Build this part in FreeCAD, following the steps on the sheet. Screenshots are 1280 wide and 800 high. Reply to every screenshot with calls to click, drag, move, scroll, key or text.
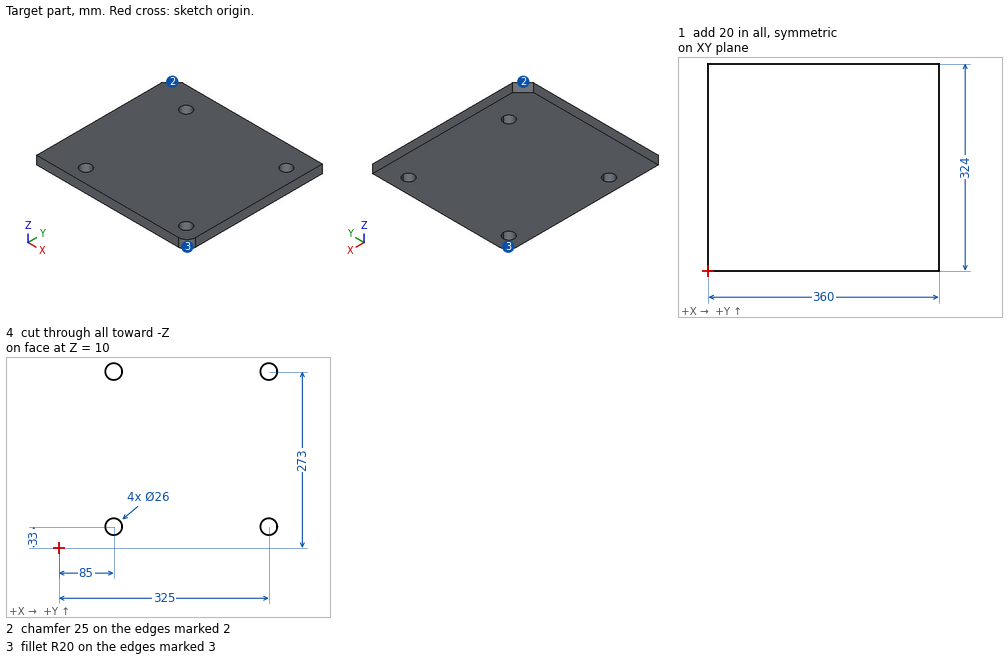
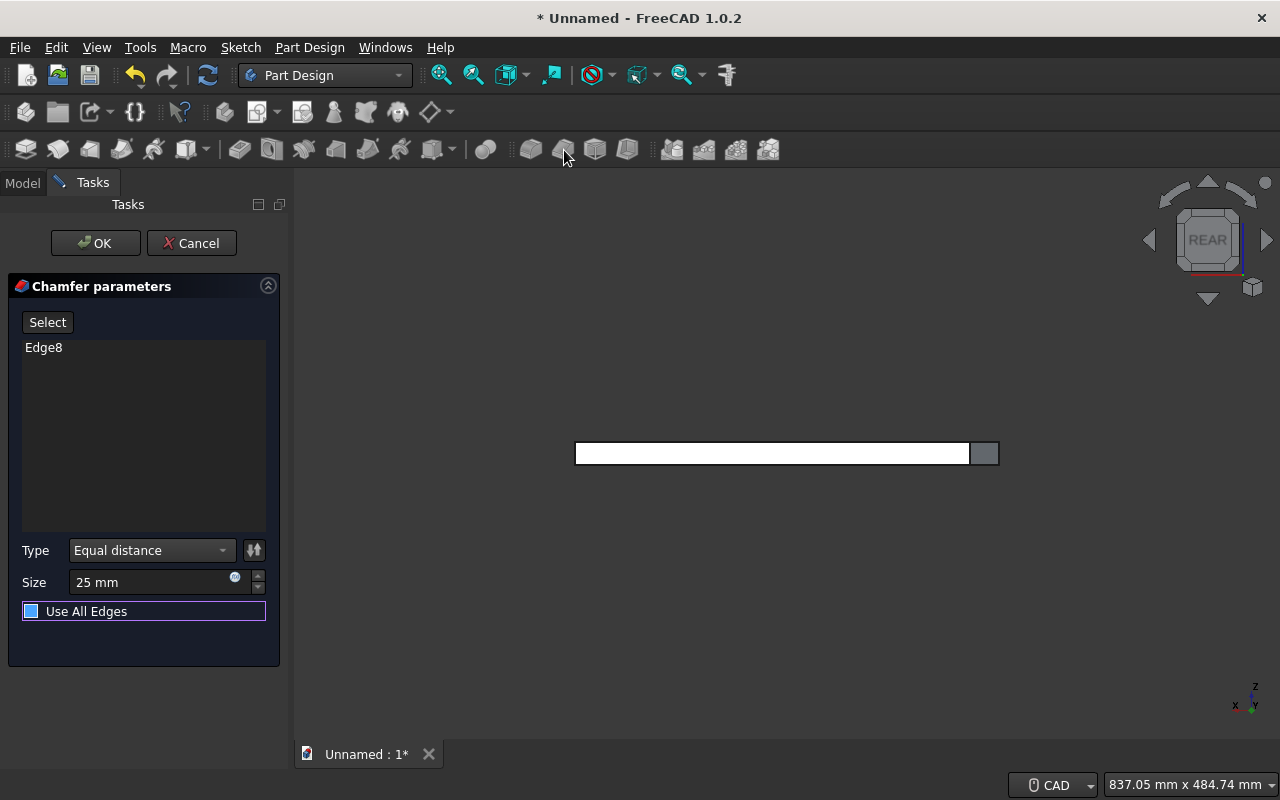
click(96, 243)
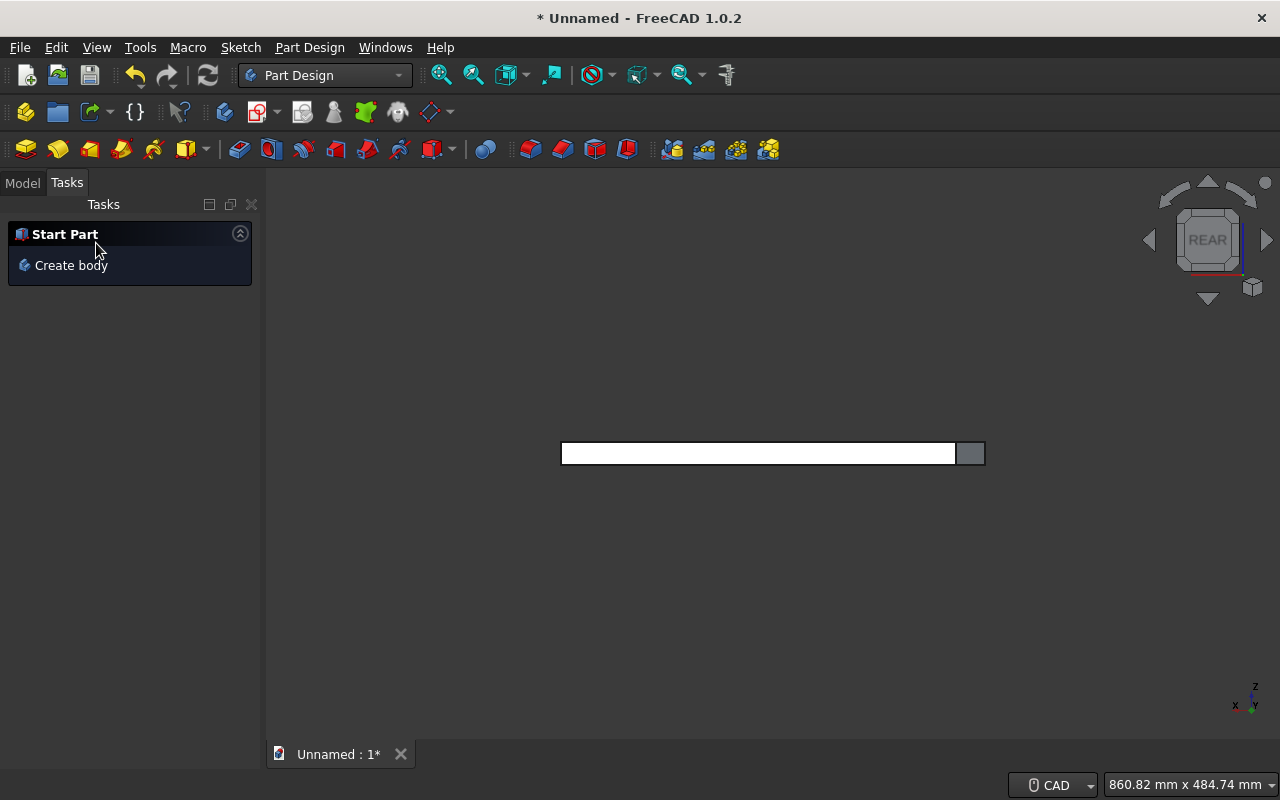
click(442, 76)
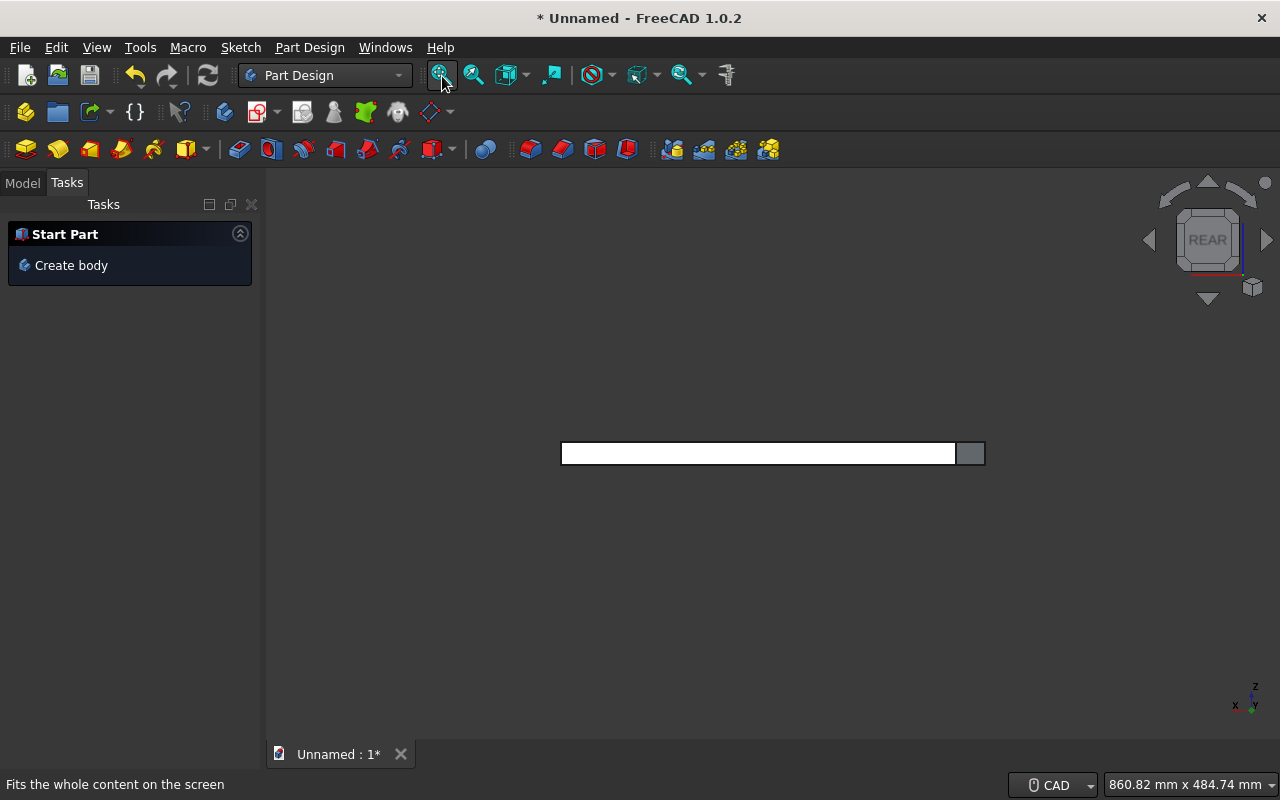
key(0)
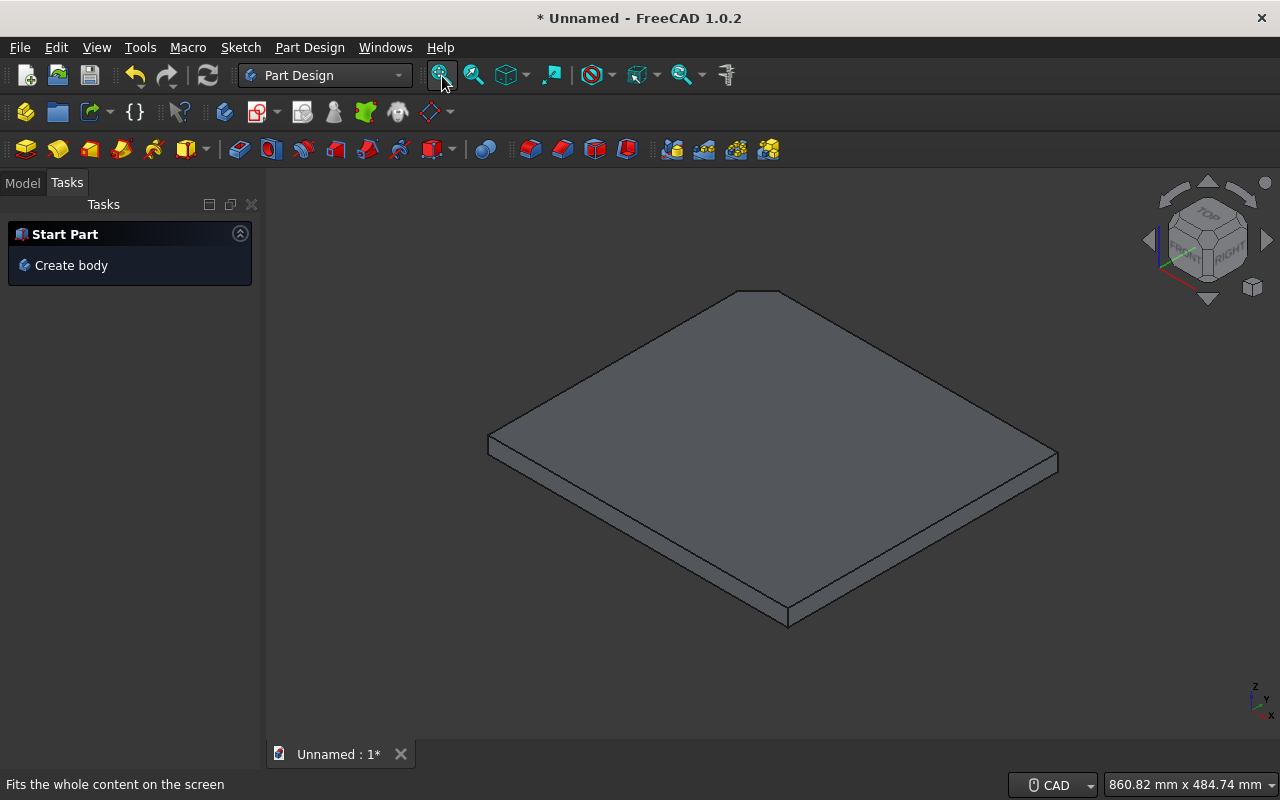
click(788, 617)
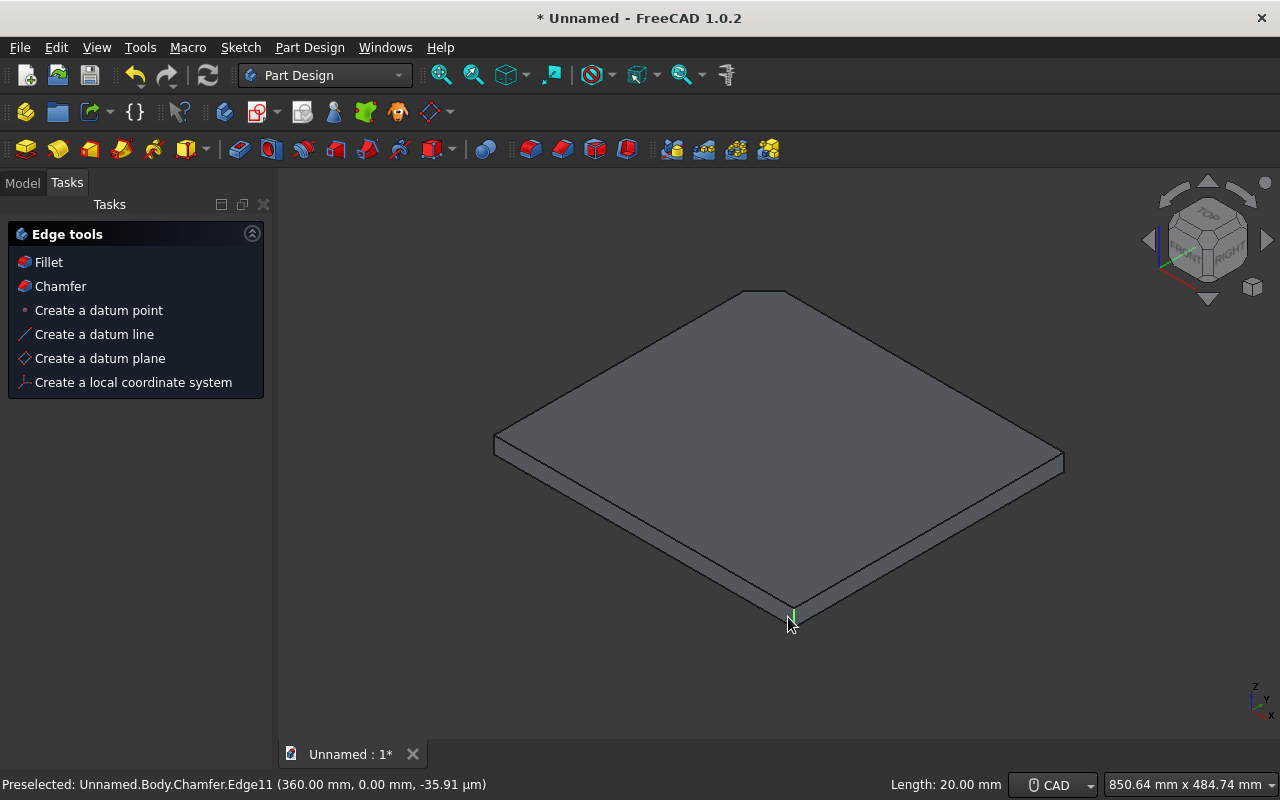
click(532, 150)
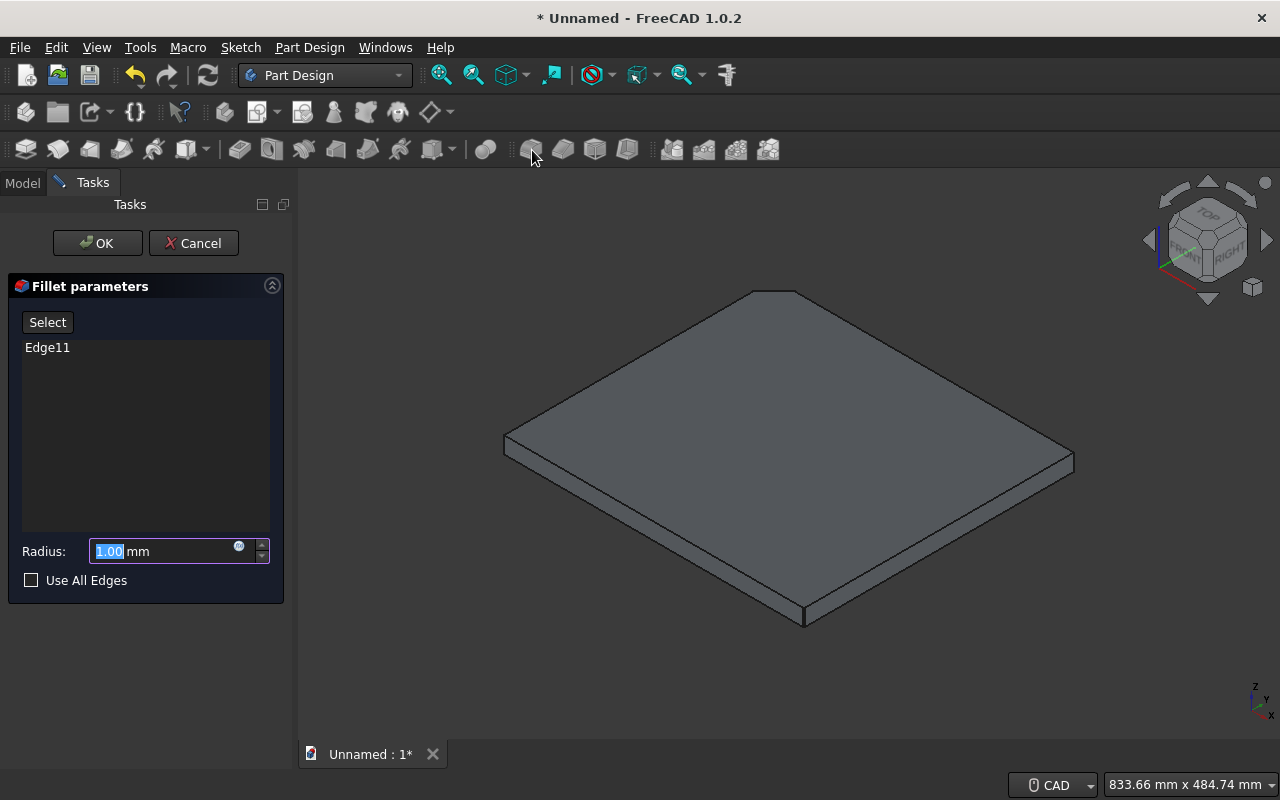
text(20)
key(Tab)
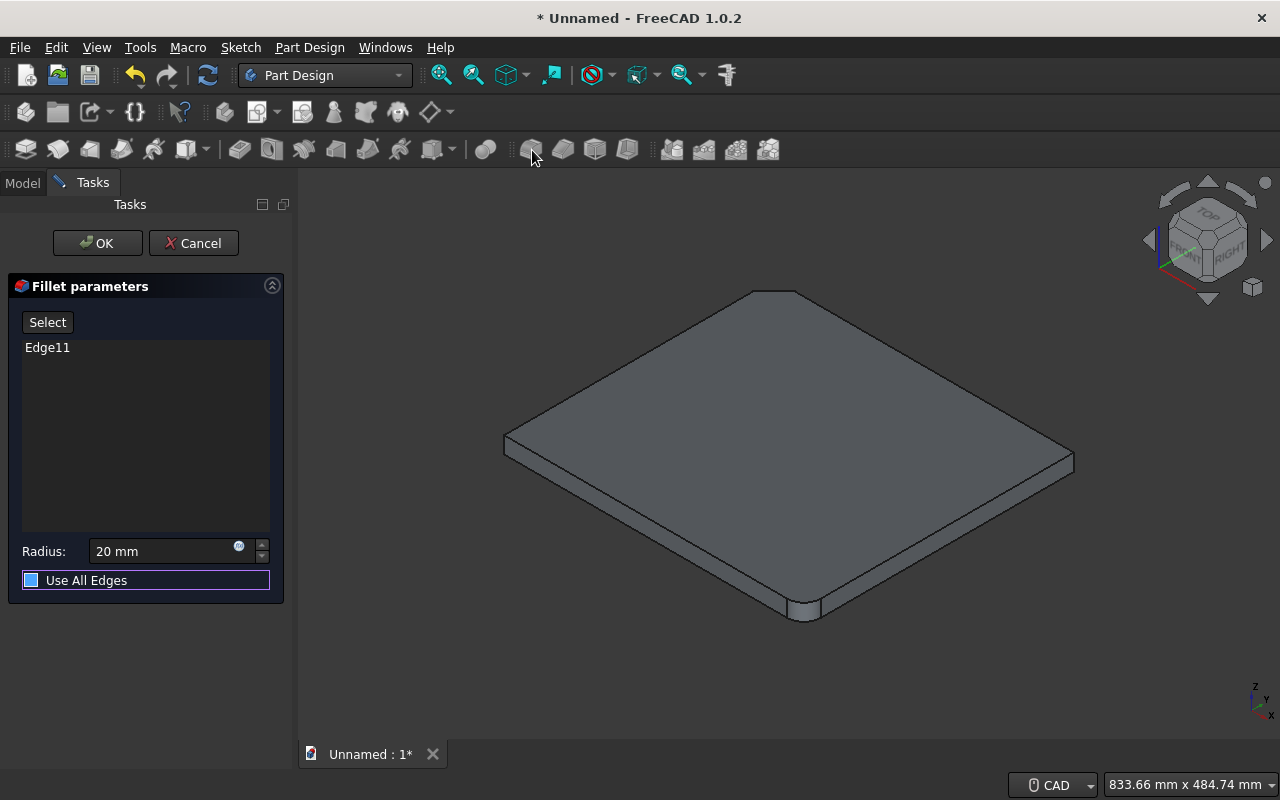
click(98, 243)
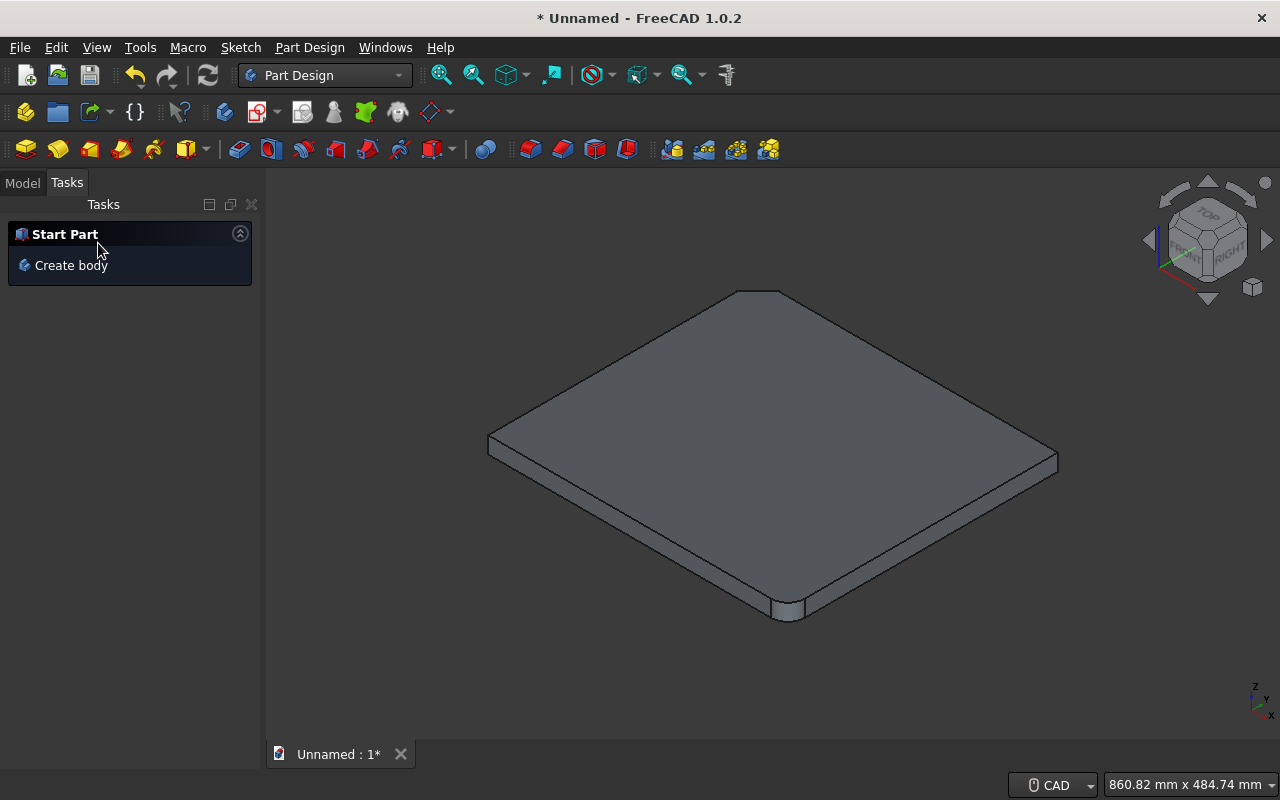
click(773, 443)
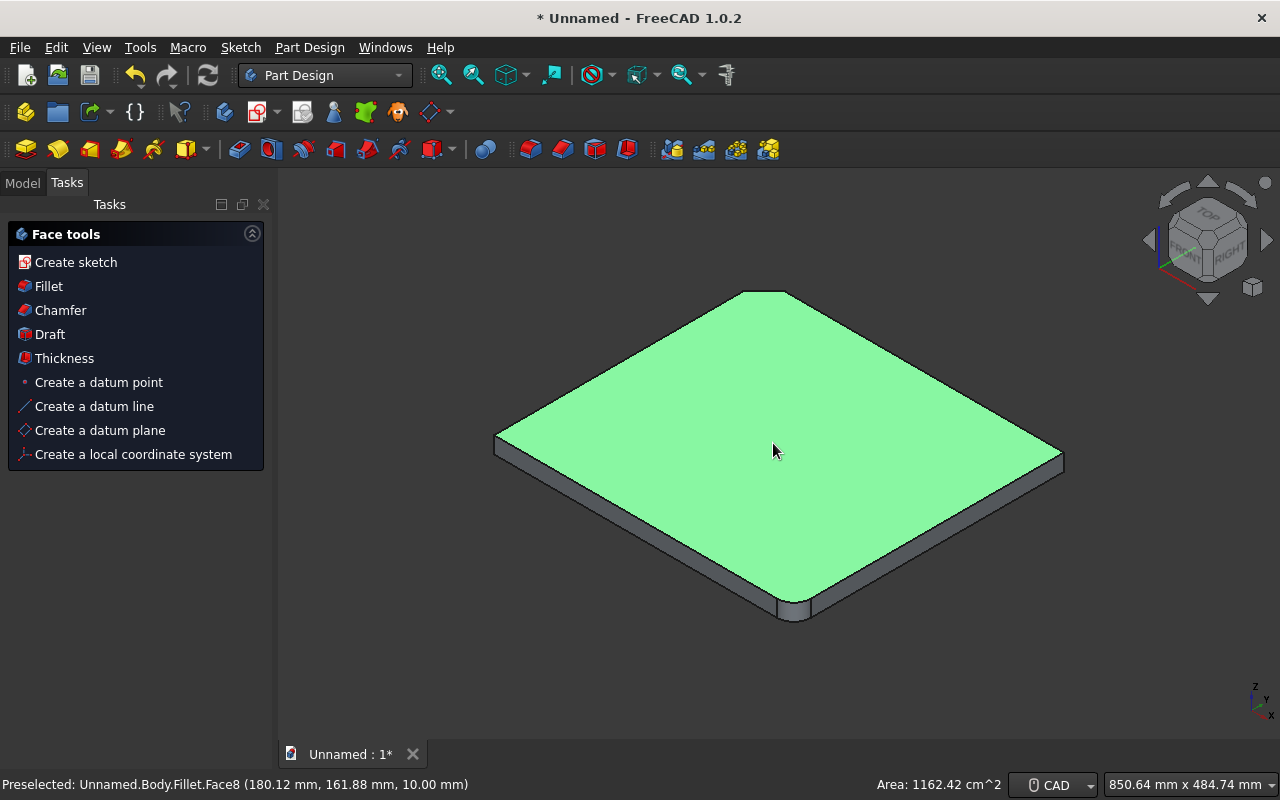
click(258, 112)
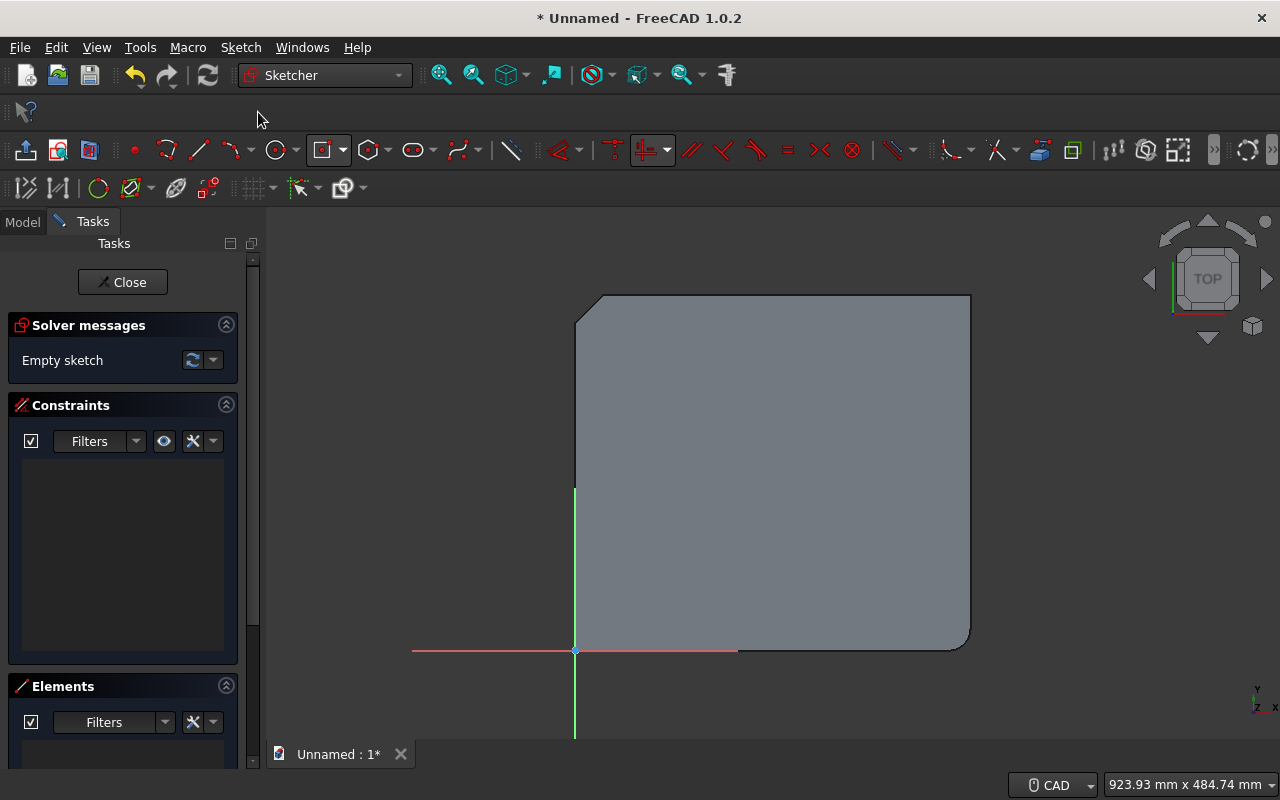
click(276, 150)